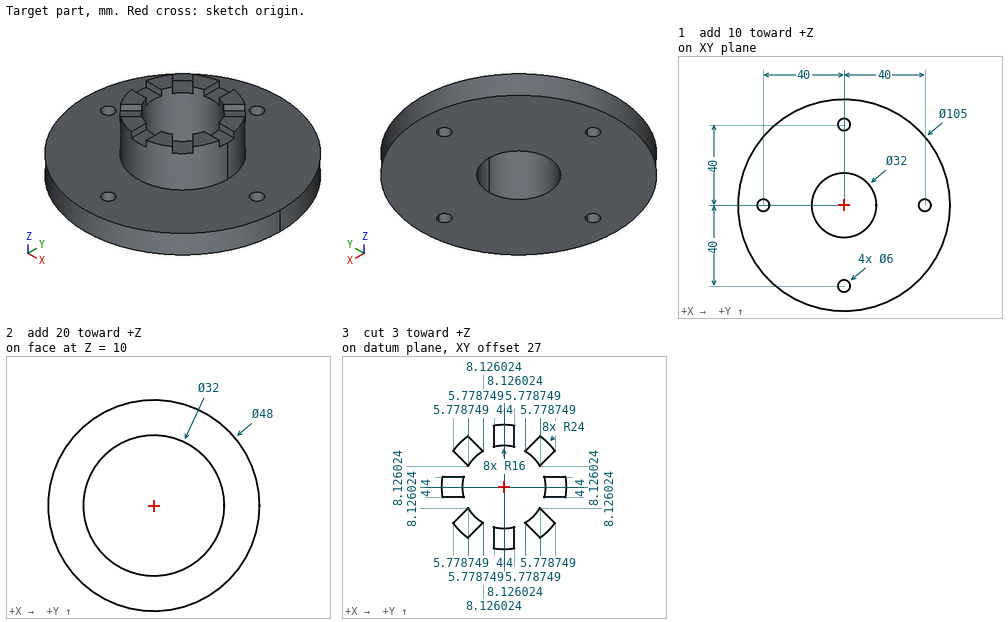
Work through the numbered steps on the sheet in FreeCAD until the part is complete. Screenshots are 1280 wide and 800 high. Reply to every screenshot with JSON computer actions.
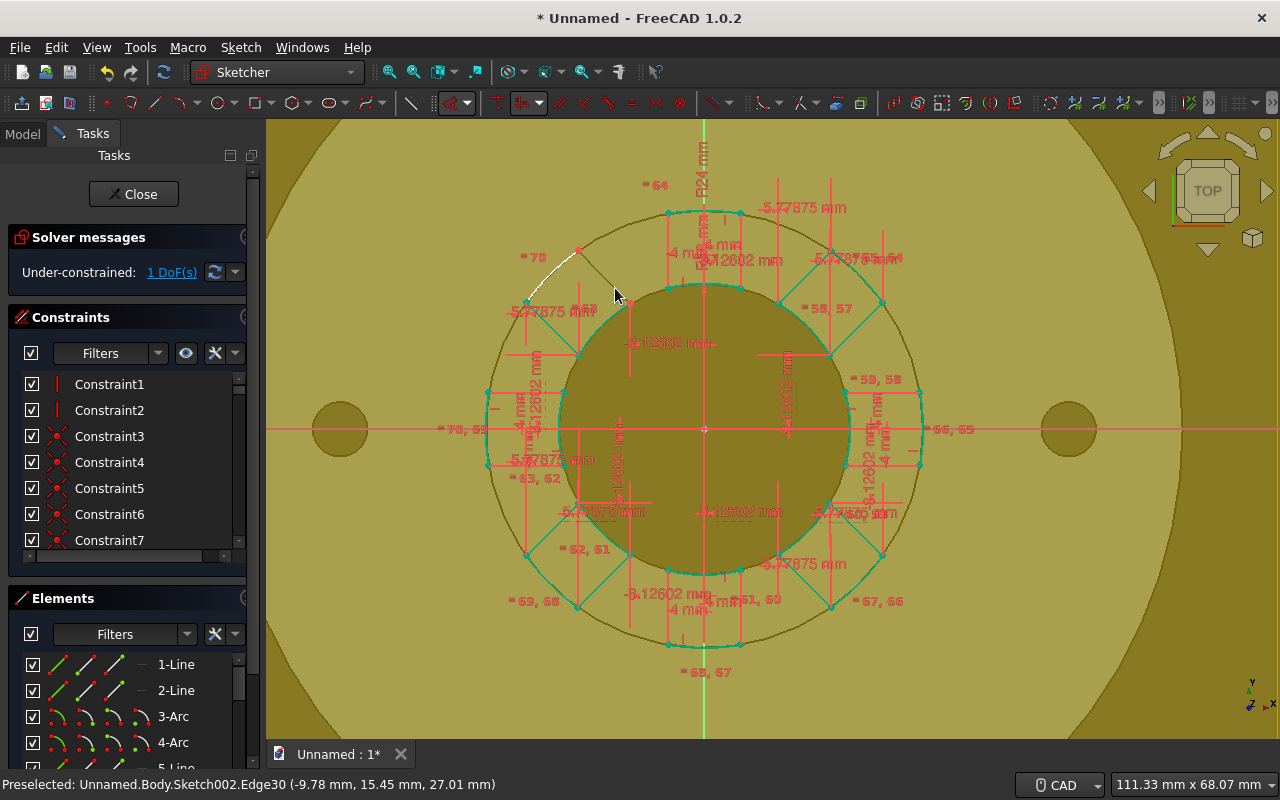
{"action": "left_click", "coordinate": [470, 104]}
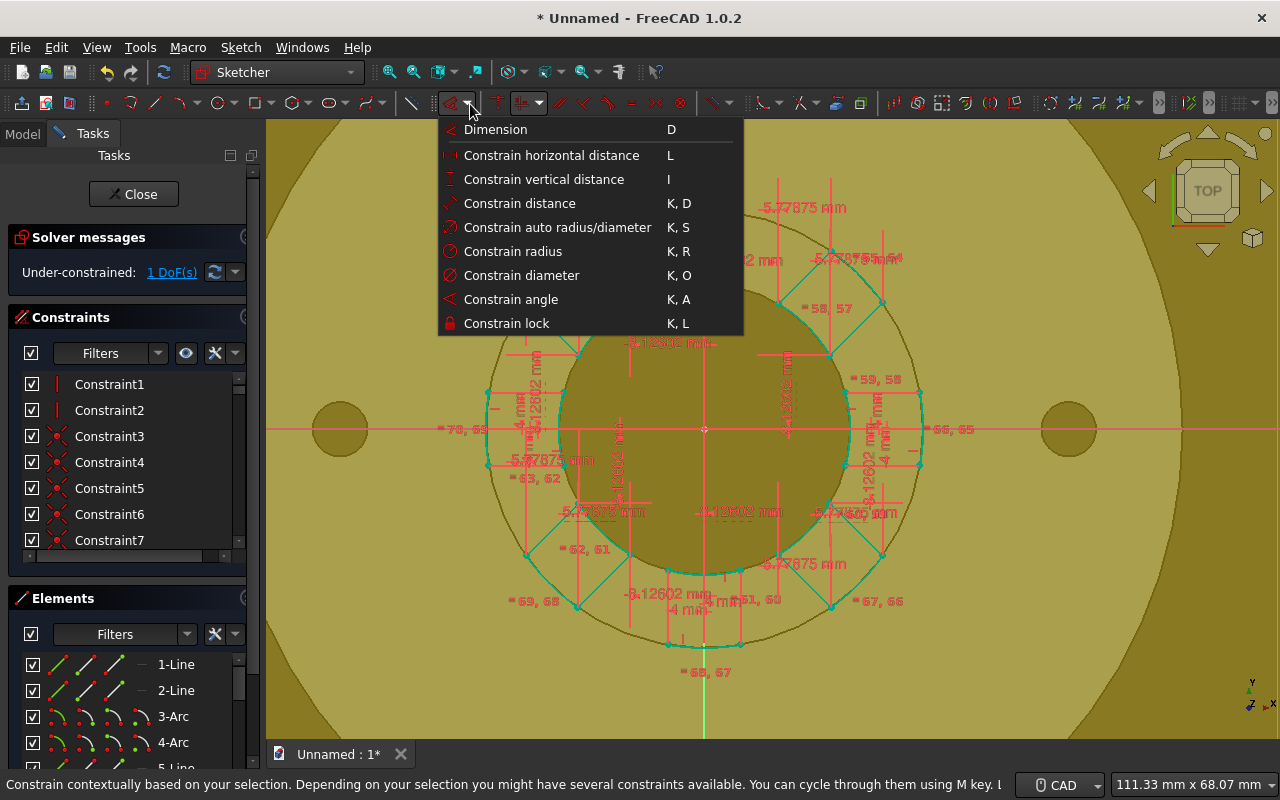
{"action": "left_click", "coordinate": [591, 155]}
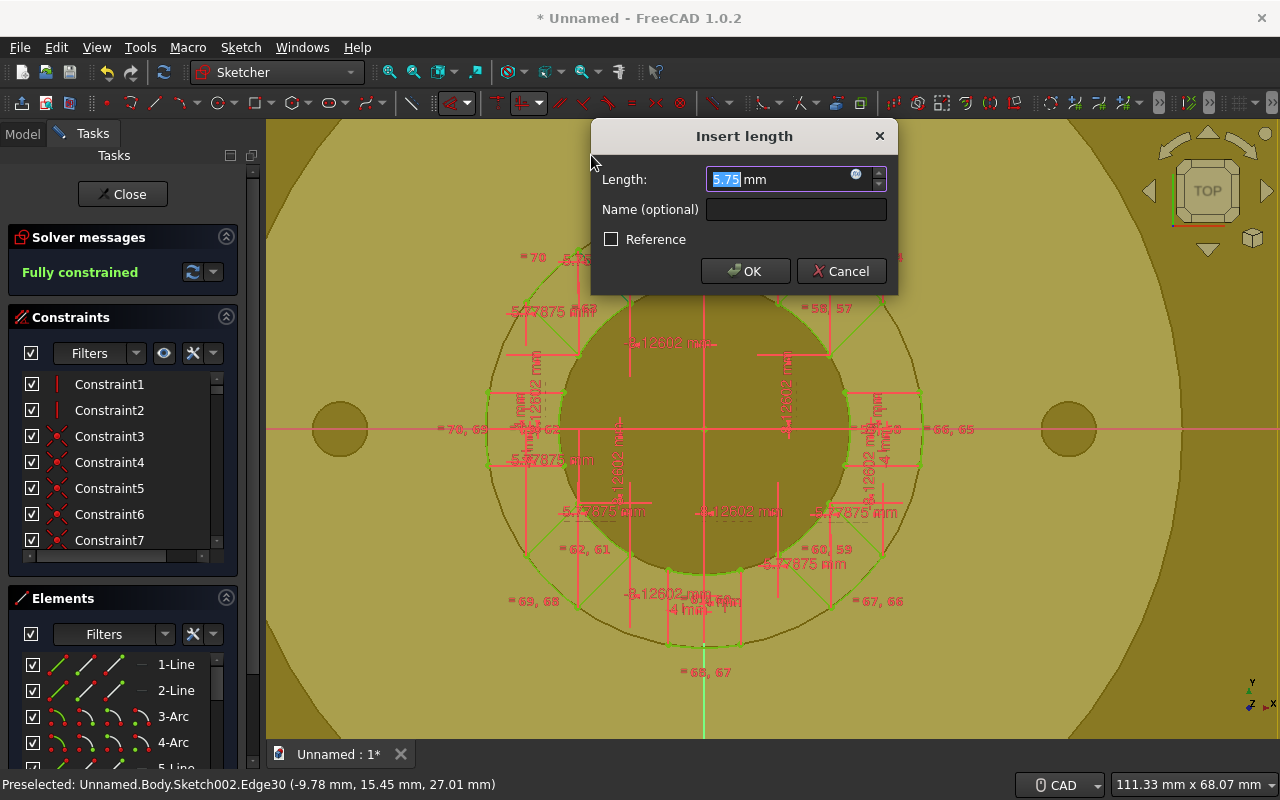
{"action": "type", "text": "5.778749"}
{"action": "key", "text": "Return"}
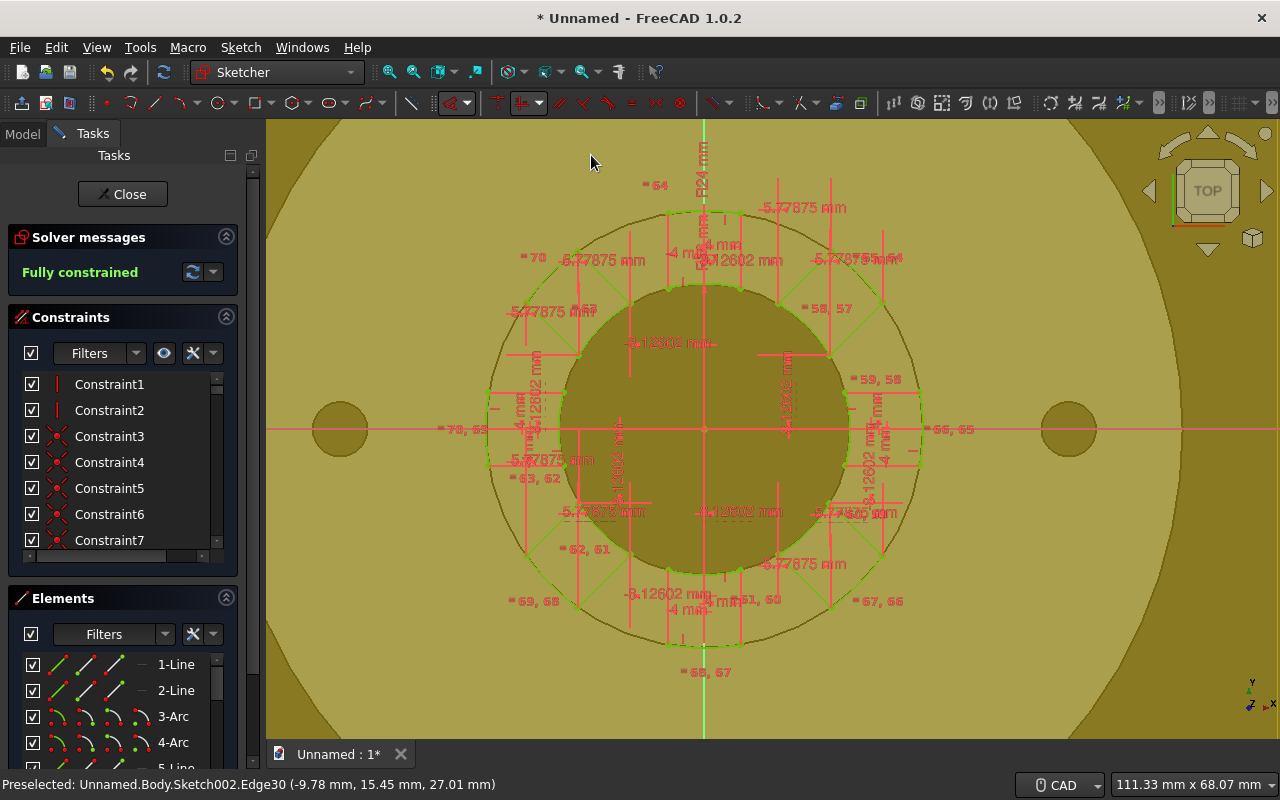
{"action": "left_click", "coordinate": [123, 194]}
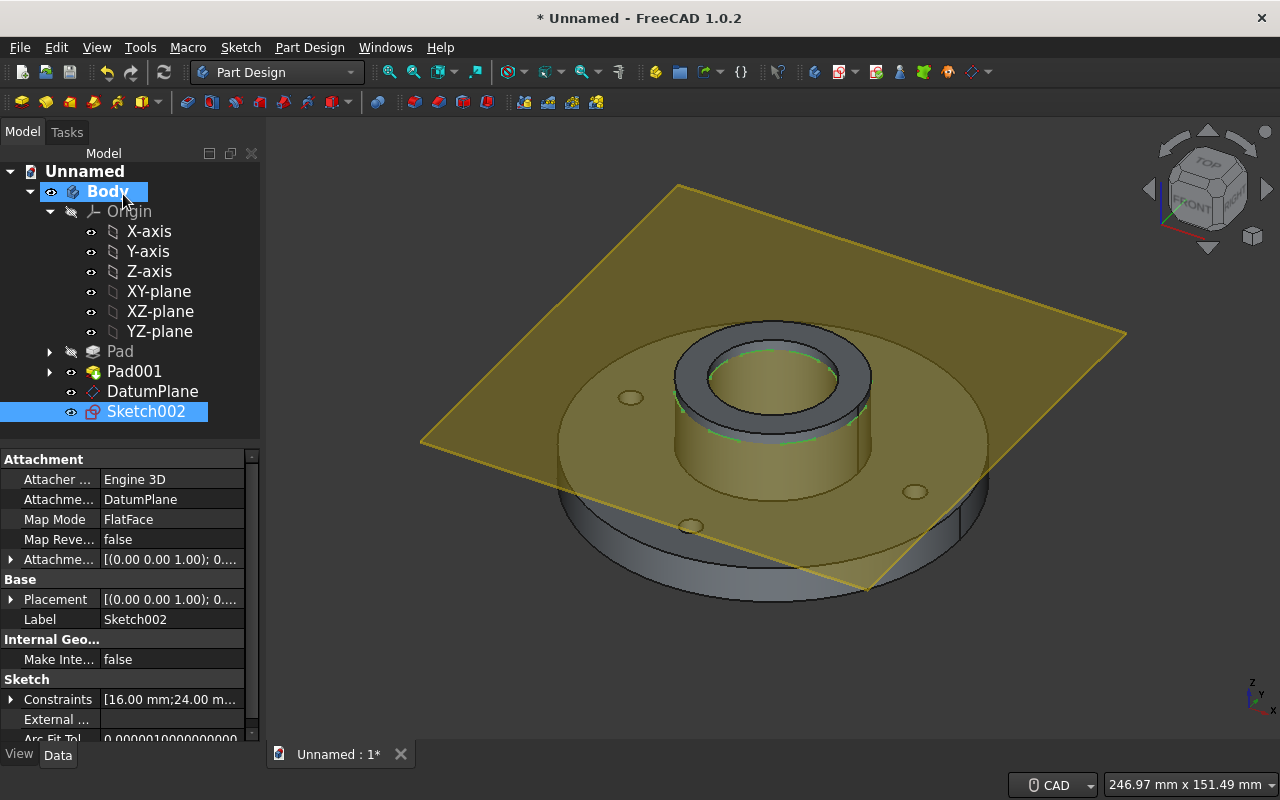
{"action": "left_click", "coordinate": [188, 102]}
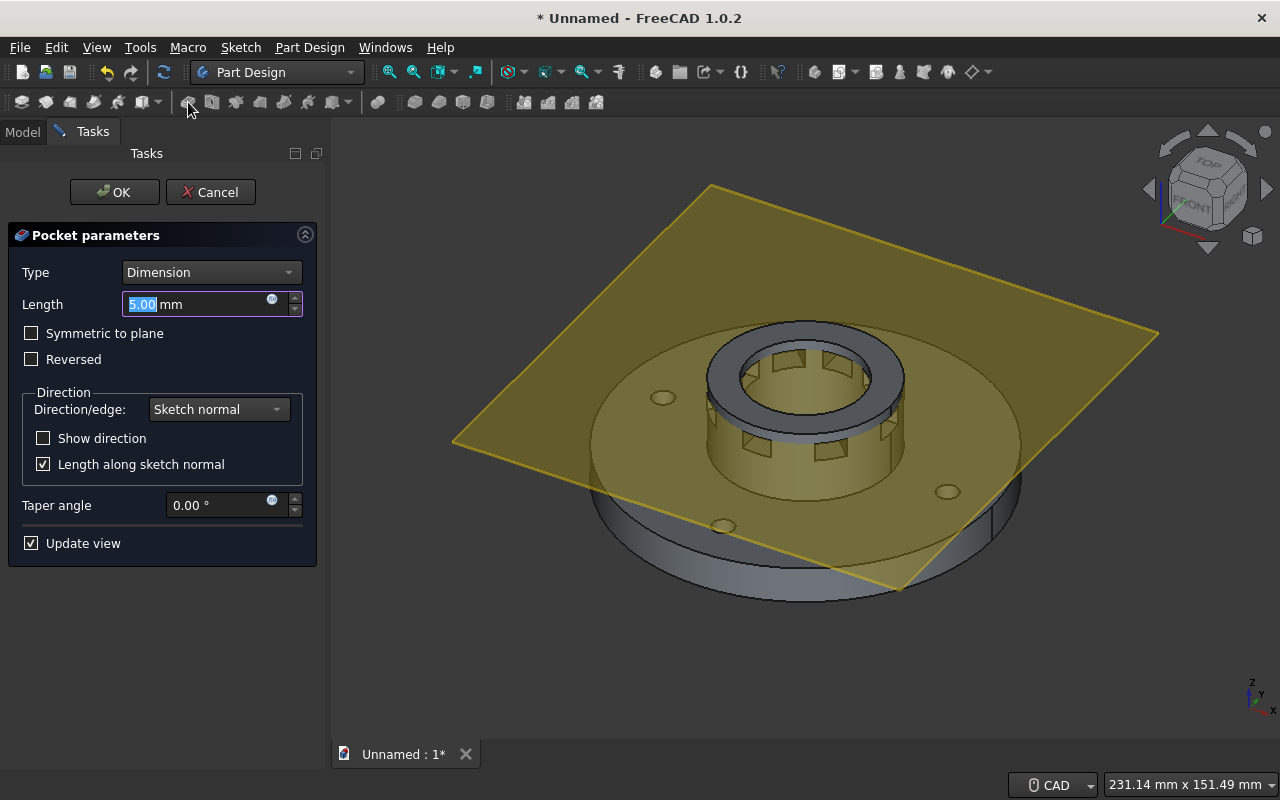
{"action": "type", "text": "3"}
{"action": "key", "text": "Tab"}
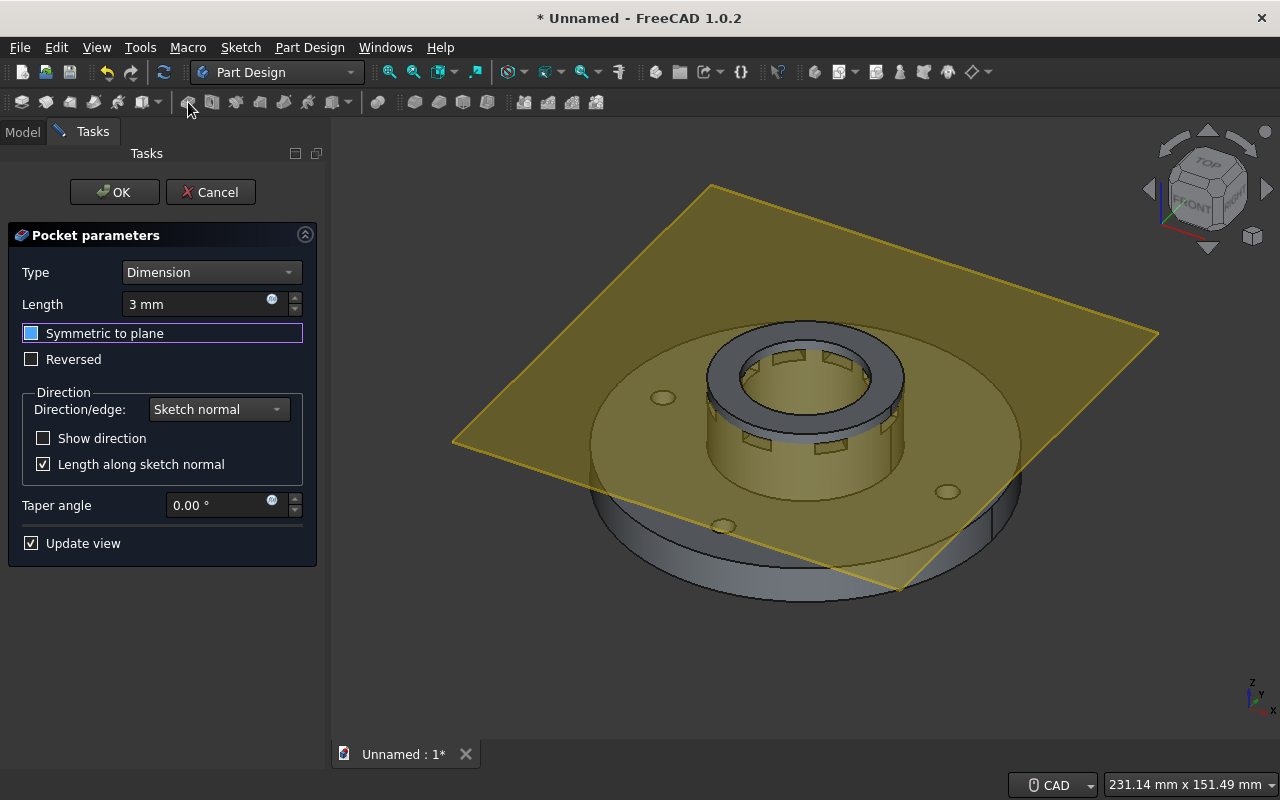
{"action": "left_click", "coordinate": [30, 359]}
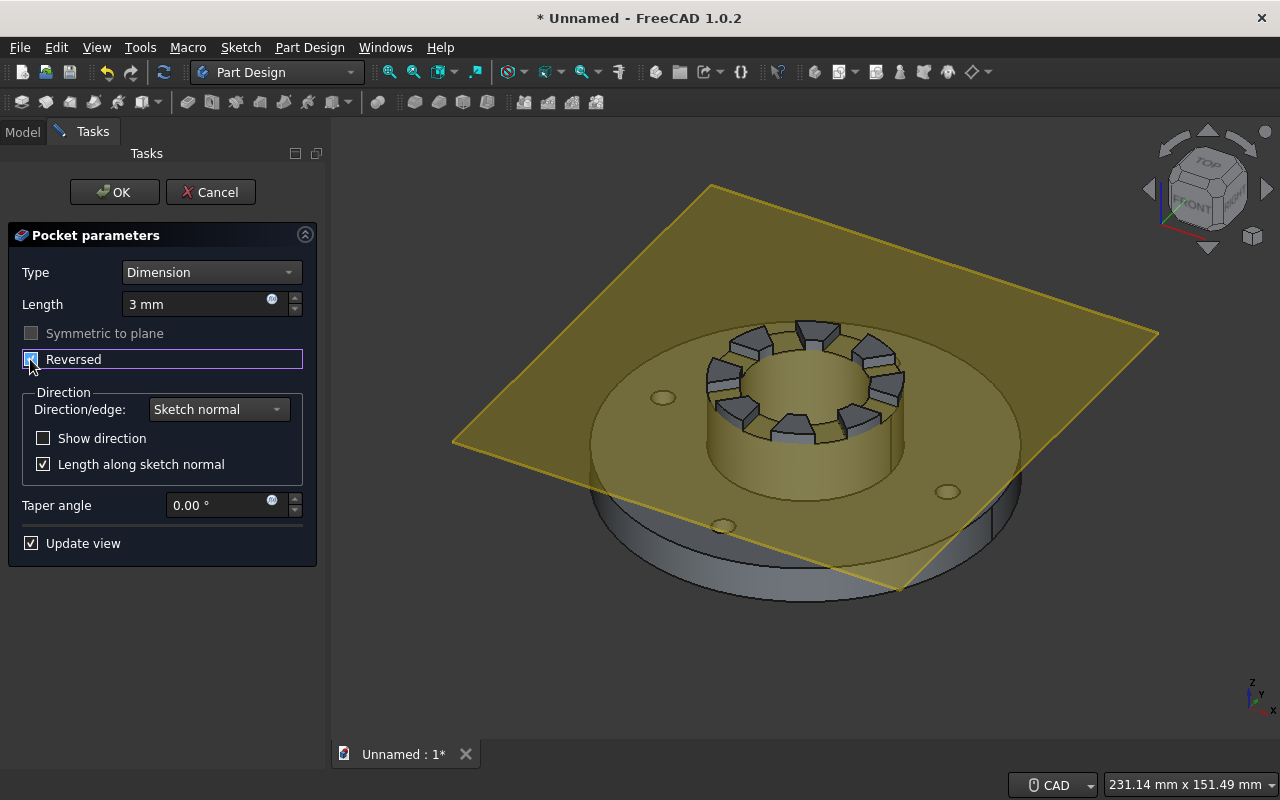
{"action": "left_click", "coordinate": [115, 192]}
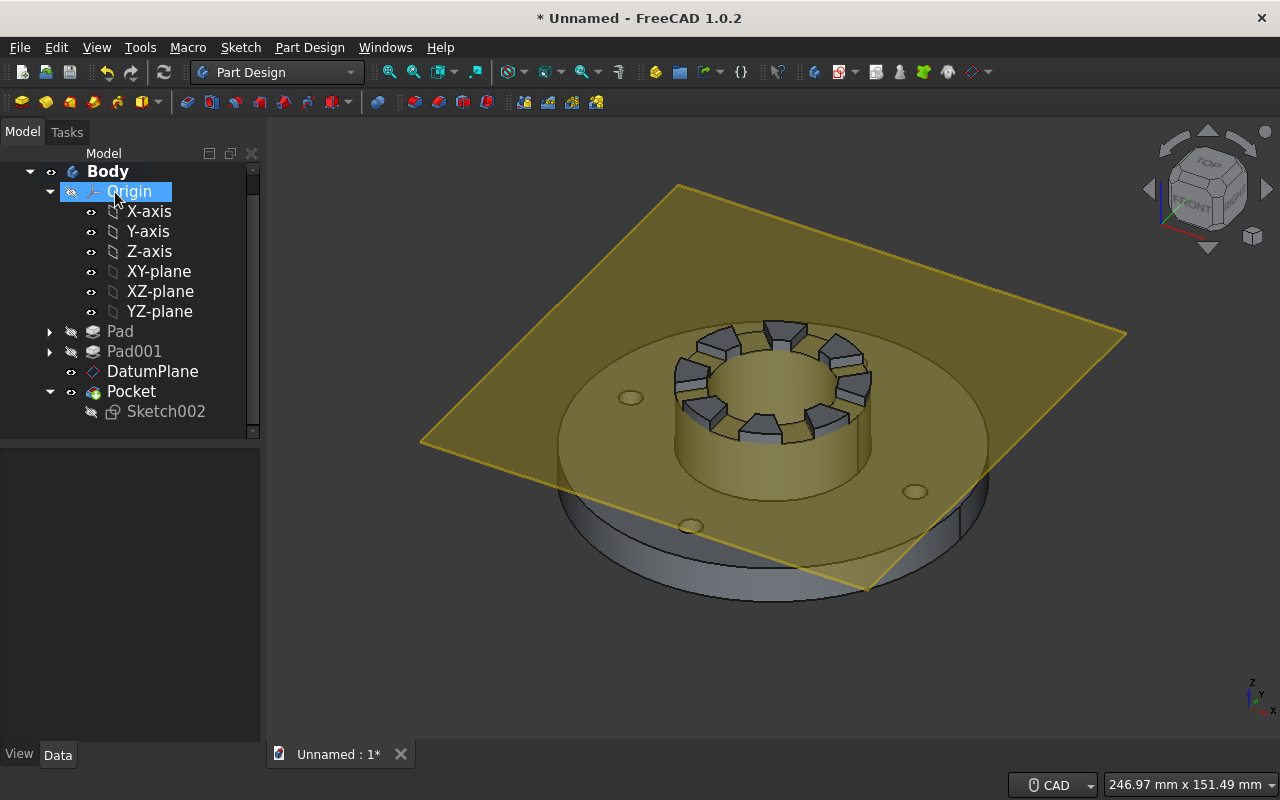
{"action": "left_click", "coordinate": [116, 372]}
{"action": "key", "text": "space"}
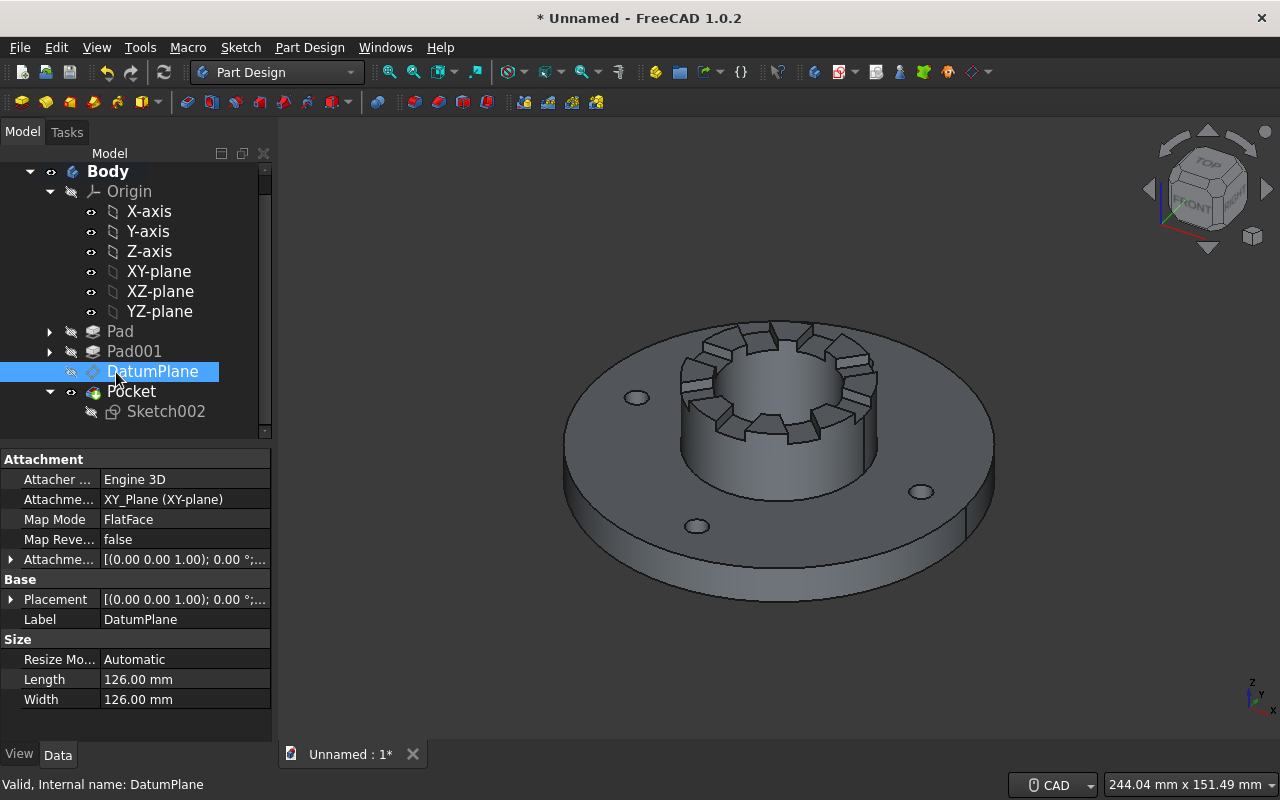
{"action": "key", "text": "0"}